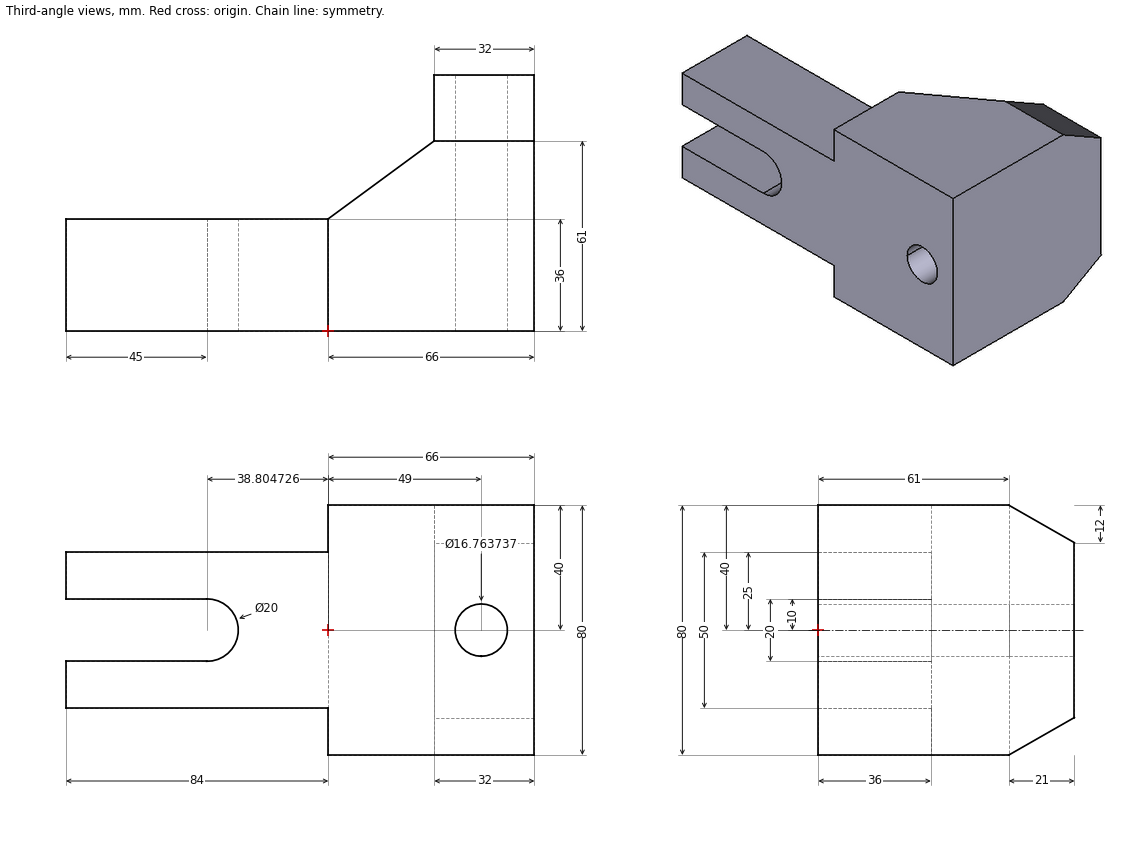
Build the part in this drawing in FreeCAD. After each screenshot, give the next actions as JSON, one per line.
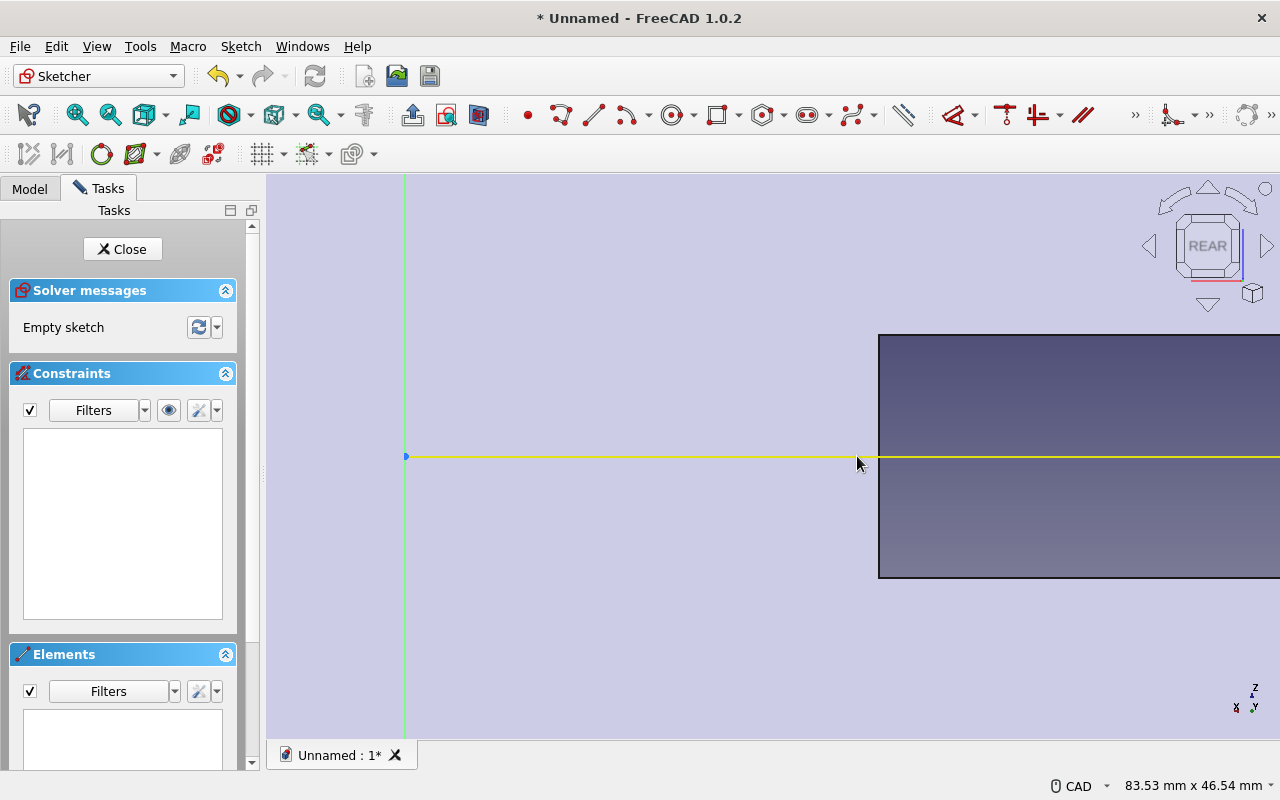
{"action": "left_click", "coordinate": [672, 116]}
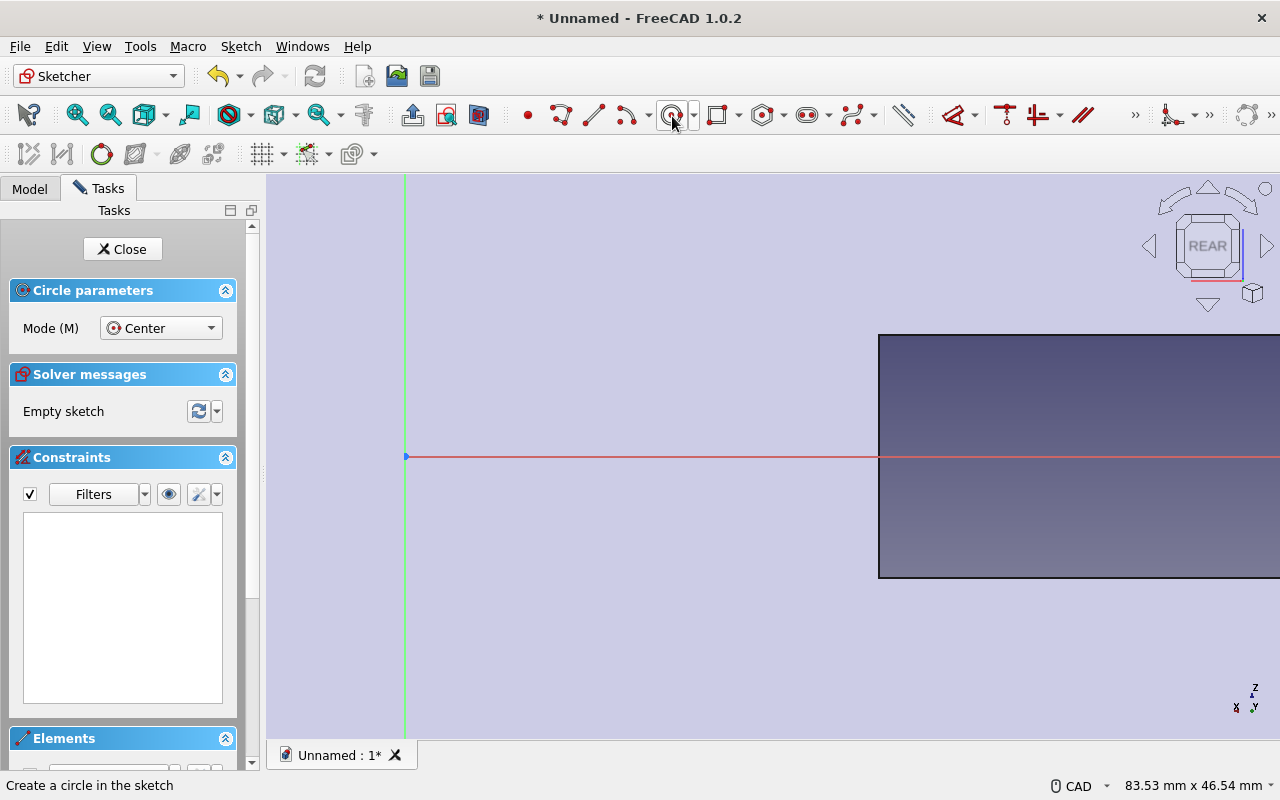
{"action": "left_click", "coordinate": [876, 456]}
{"action": "left_click", "coordinate": [962, 371]}
{"action": "key", "text": "Escape"}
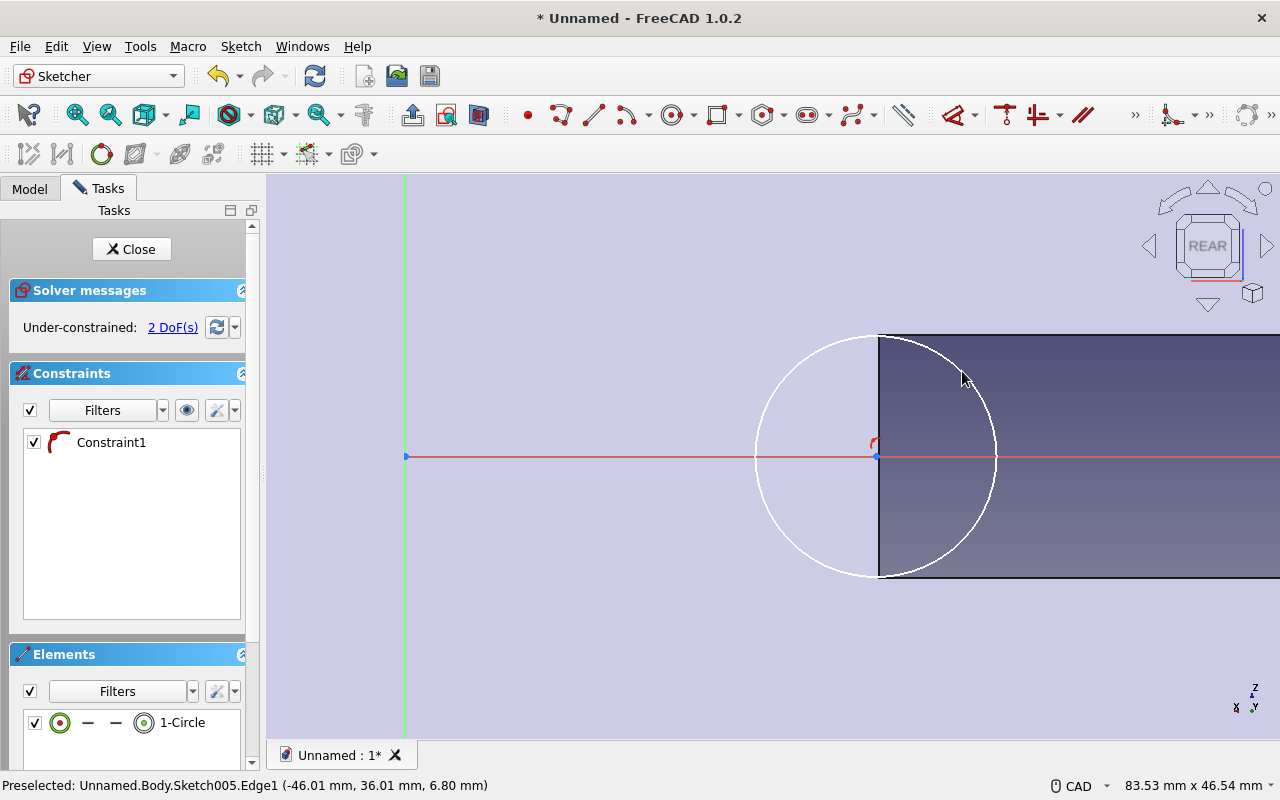
{"action": "key", "text": "d"}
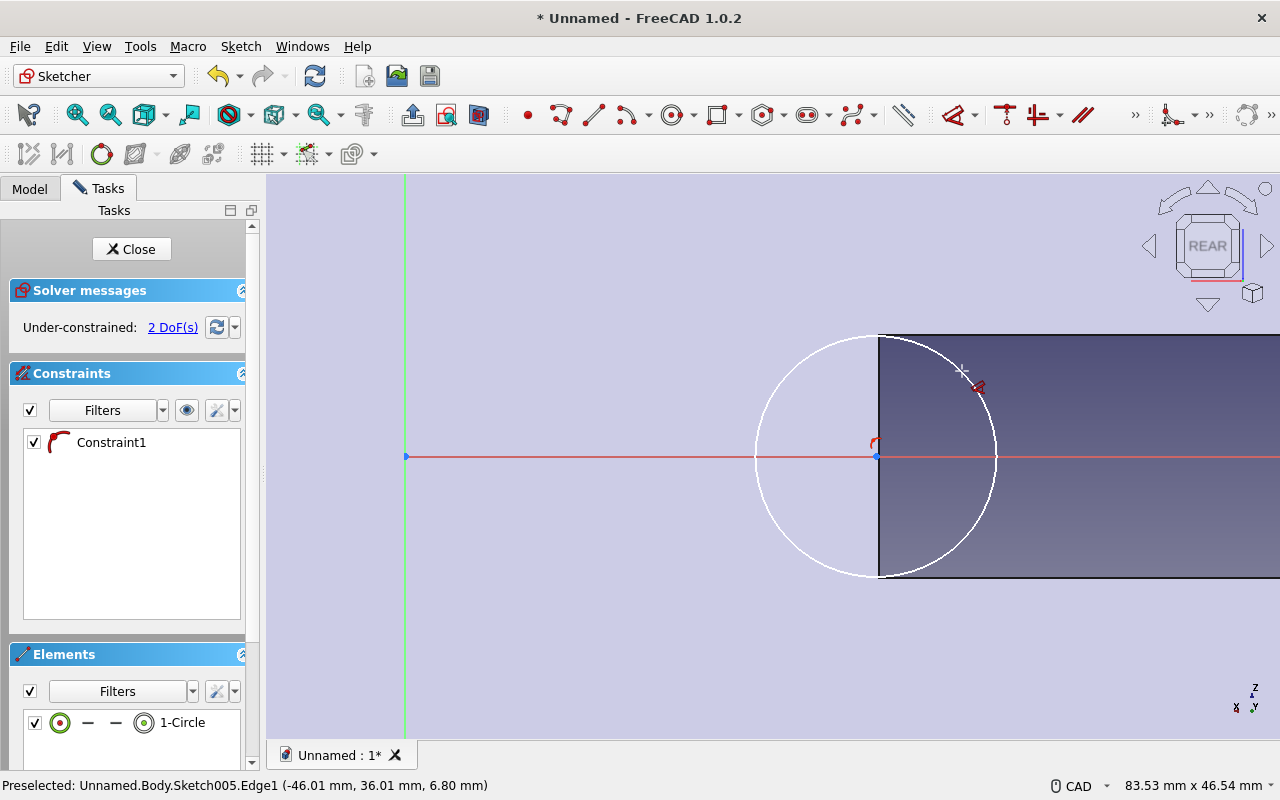
{"action": "left_click", "coordinate": [961, 371]}
{"action": "left_click", "coordinate": [984, 348]}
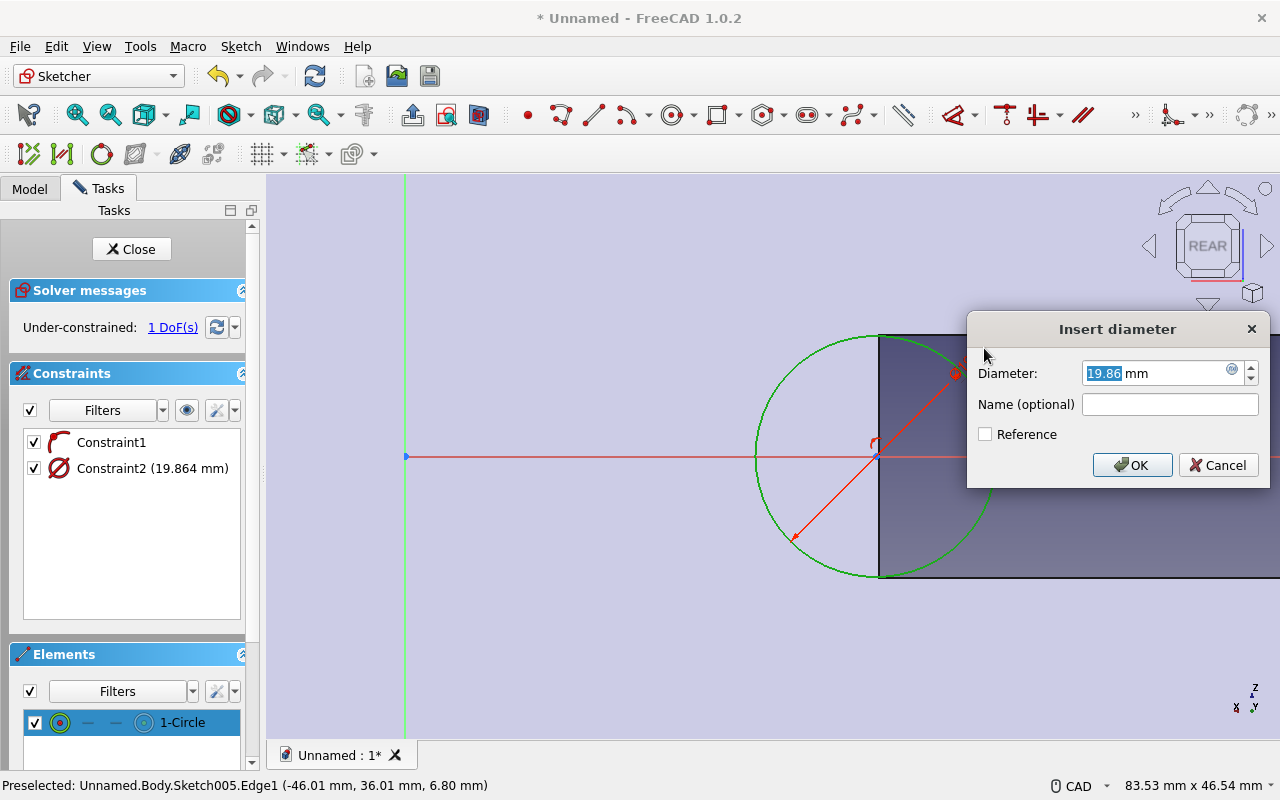
{"action": "type", "text": "20"}
{"action": "key", "text": "Return"}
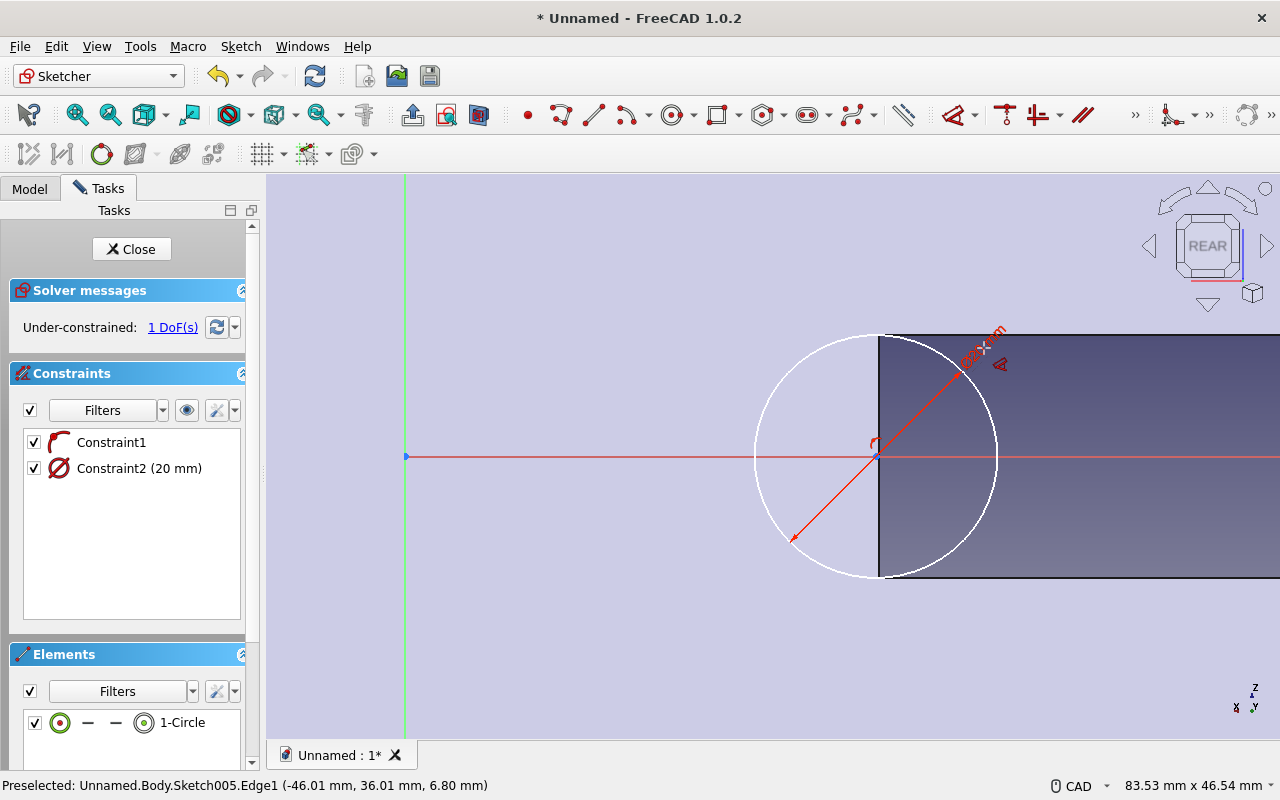
{"action": "left_click", "coordinate": [876, 456]}
{"action": "left_click", "coordinate": [641, 490]}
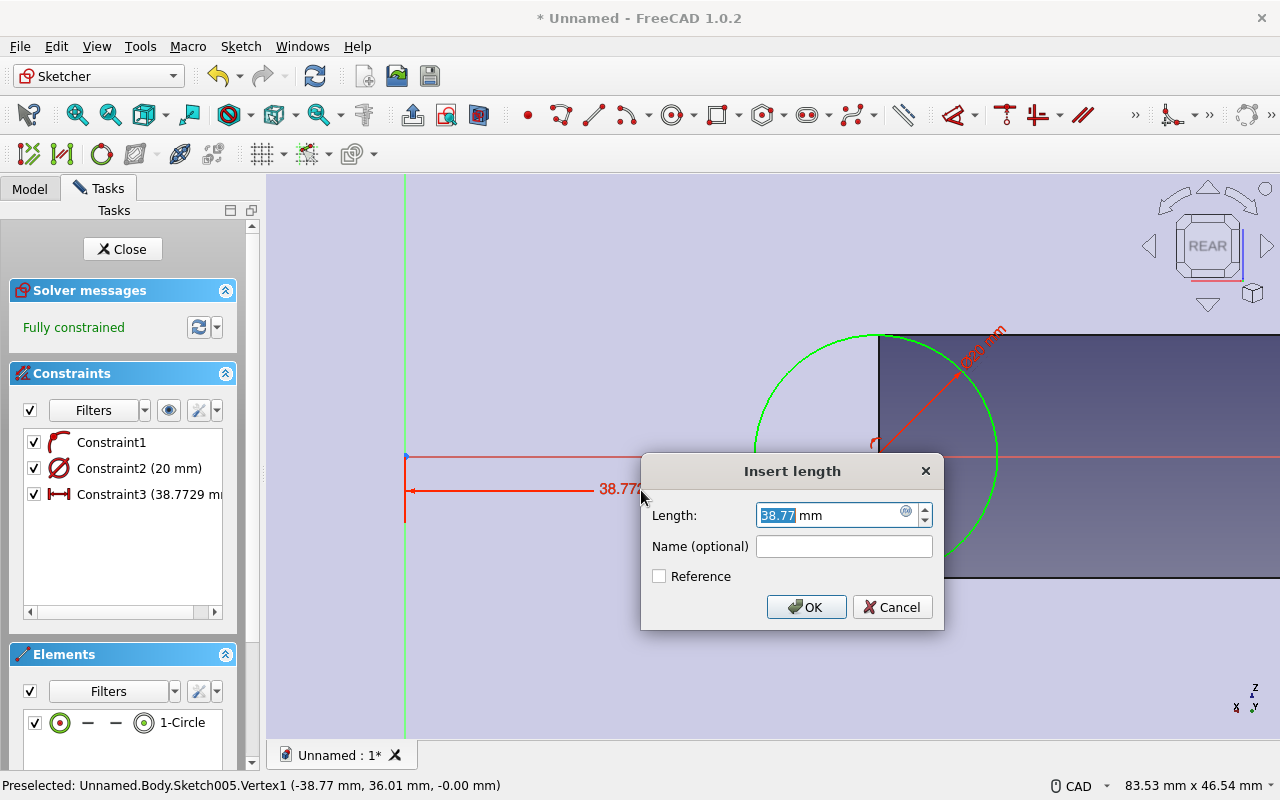
{"action": "type", "text": "38.804726"}
{"action": "key", "text": "Return"}
{"action": "key", "text": "Escape"}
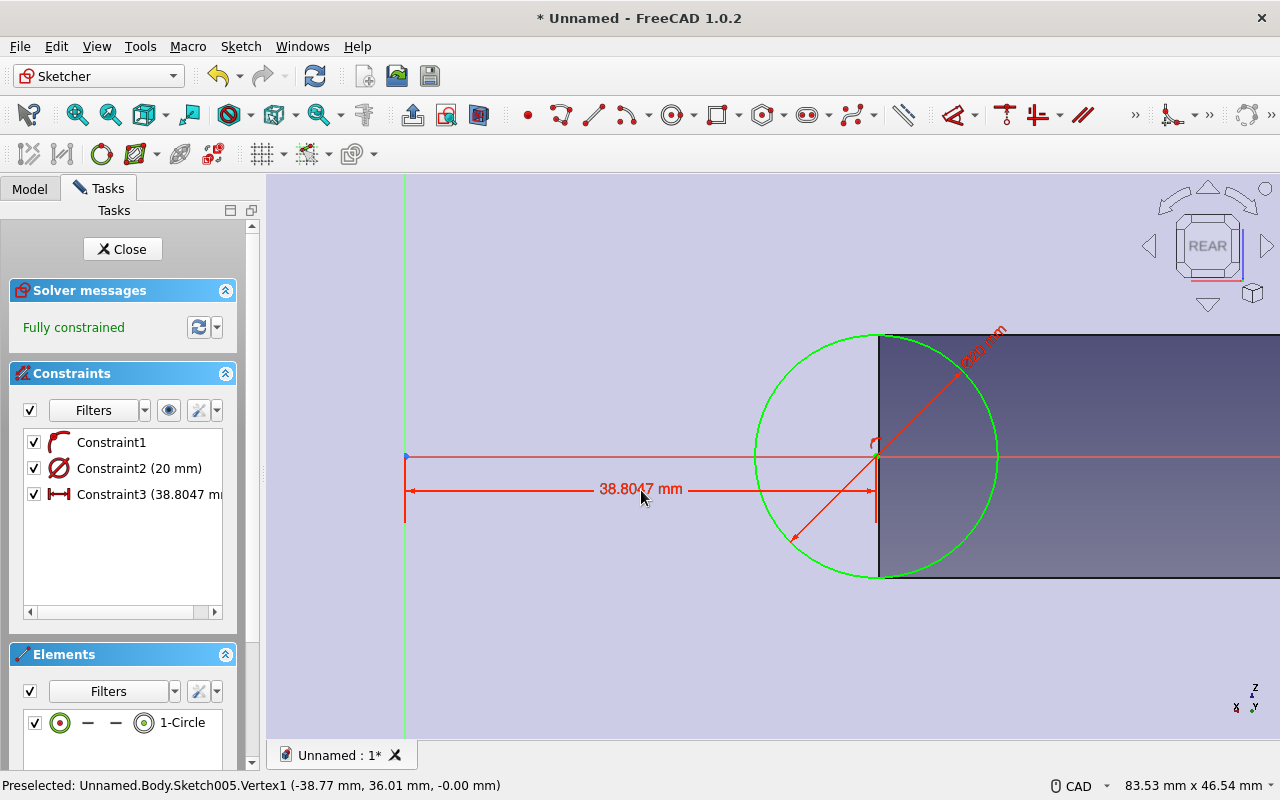
{"action": "left_click", "coordinate": [123, 249]}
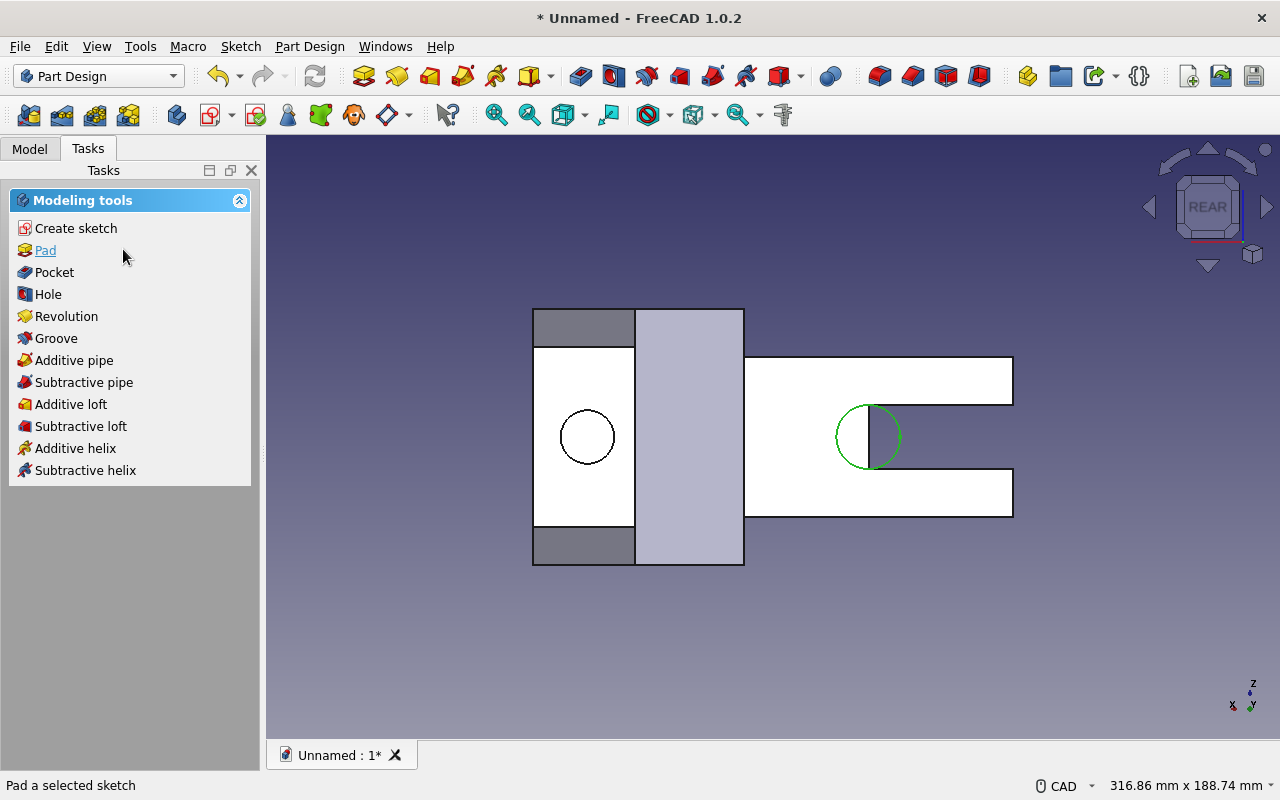
{"action": "left_click", "coordinate": [581, 76]}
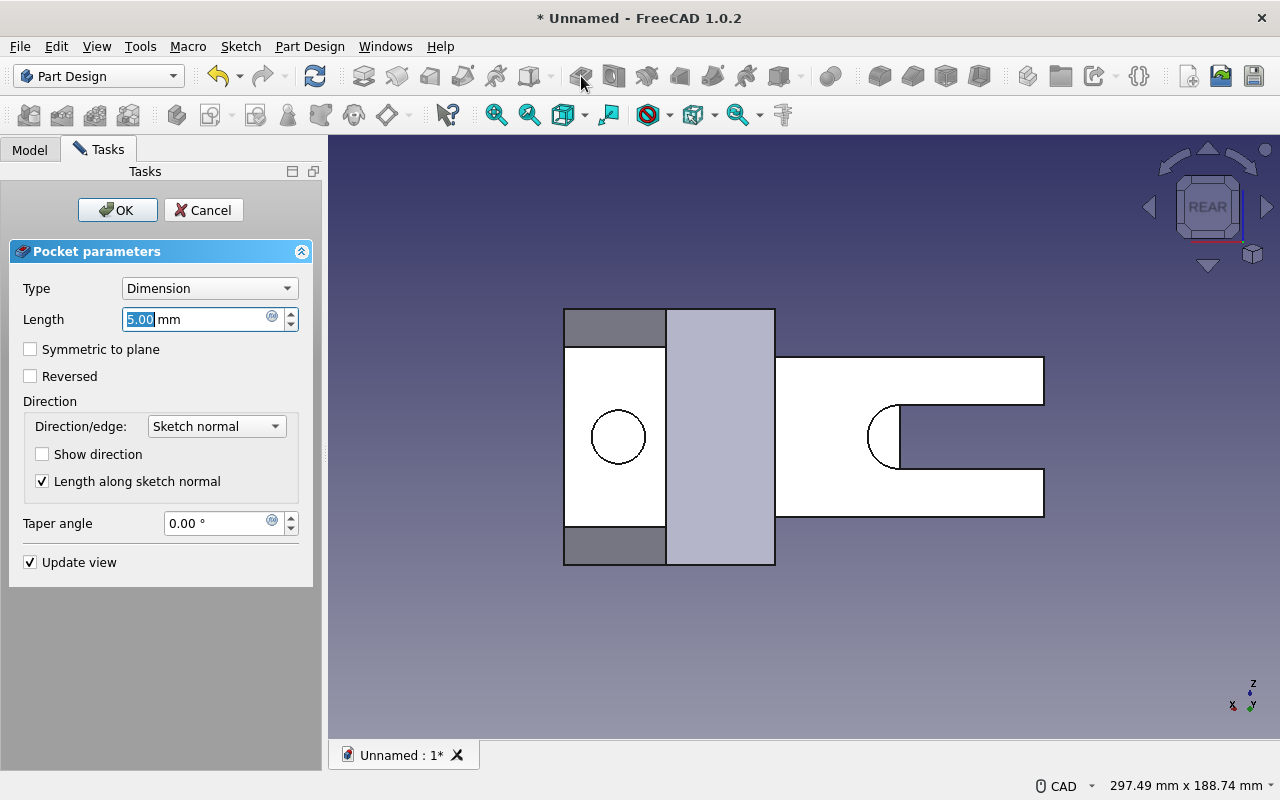
{"action": "type", "text": "36"}
{"action": "key", "text": "Tab"}